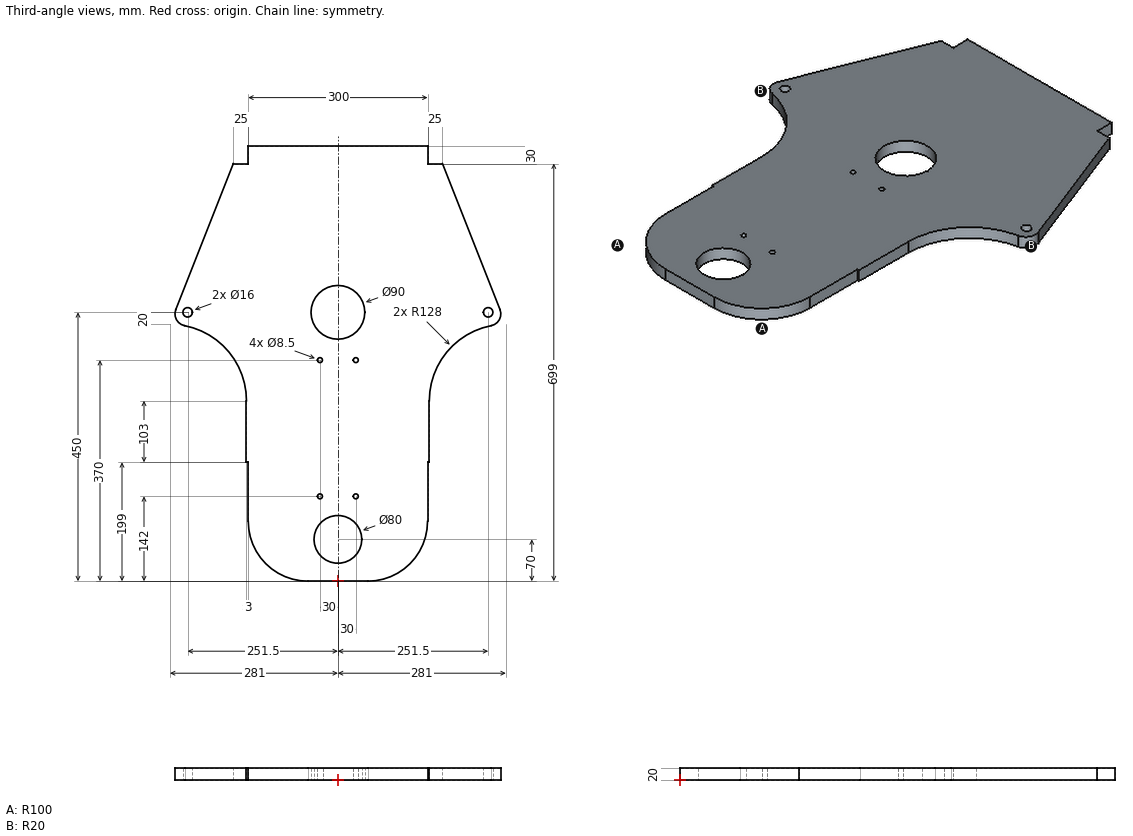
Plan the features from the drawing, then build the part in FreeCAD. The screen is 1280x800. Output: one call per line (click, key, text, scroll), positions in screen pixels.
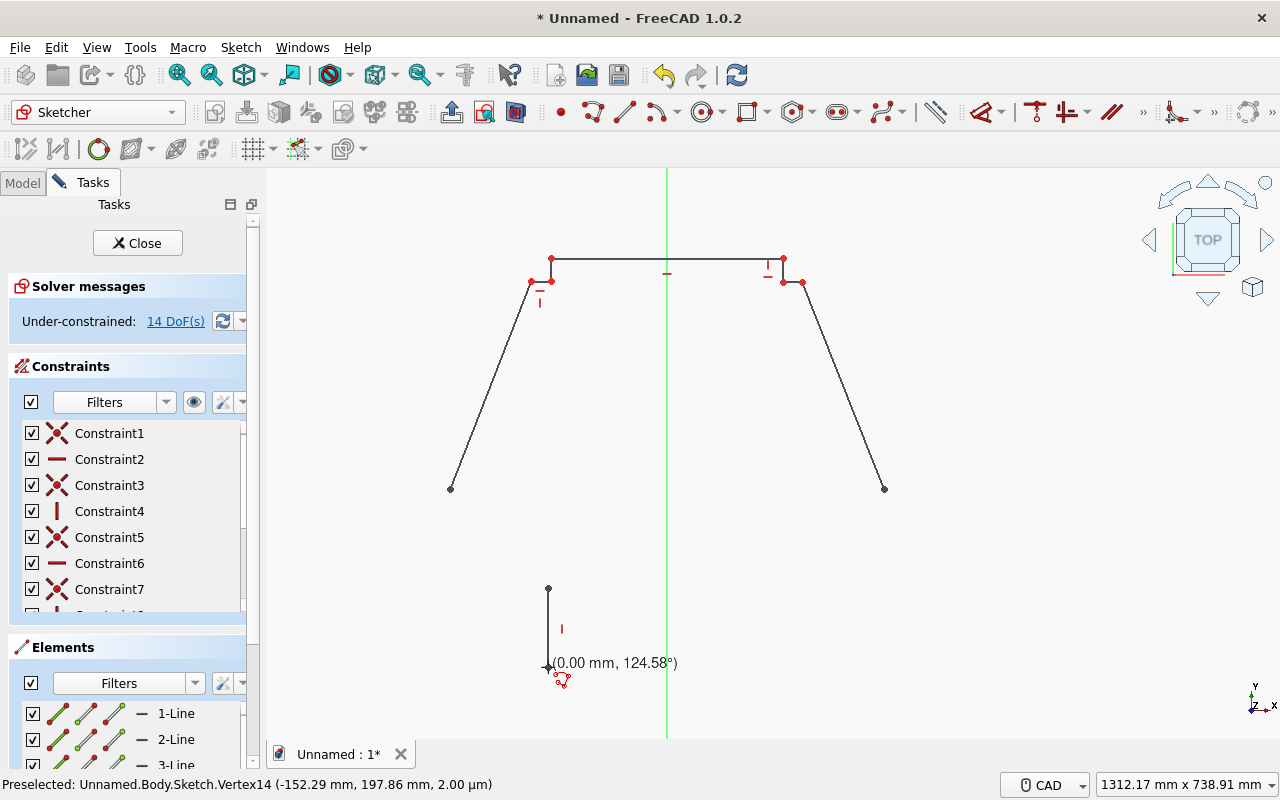
scroll(551, 667, up, 10)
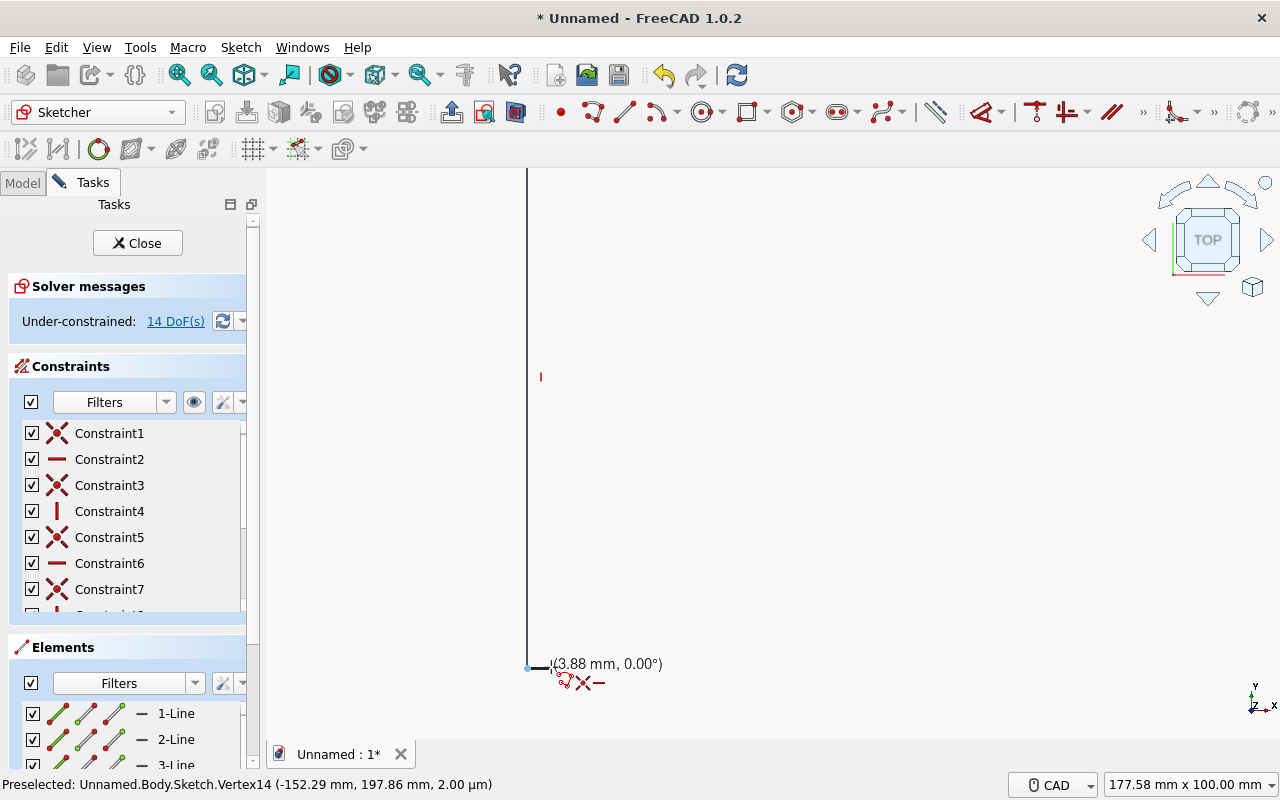
click(547, 661)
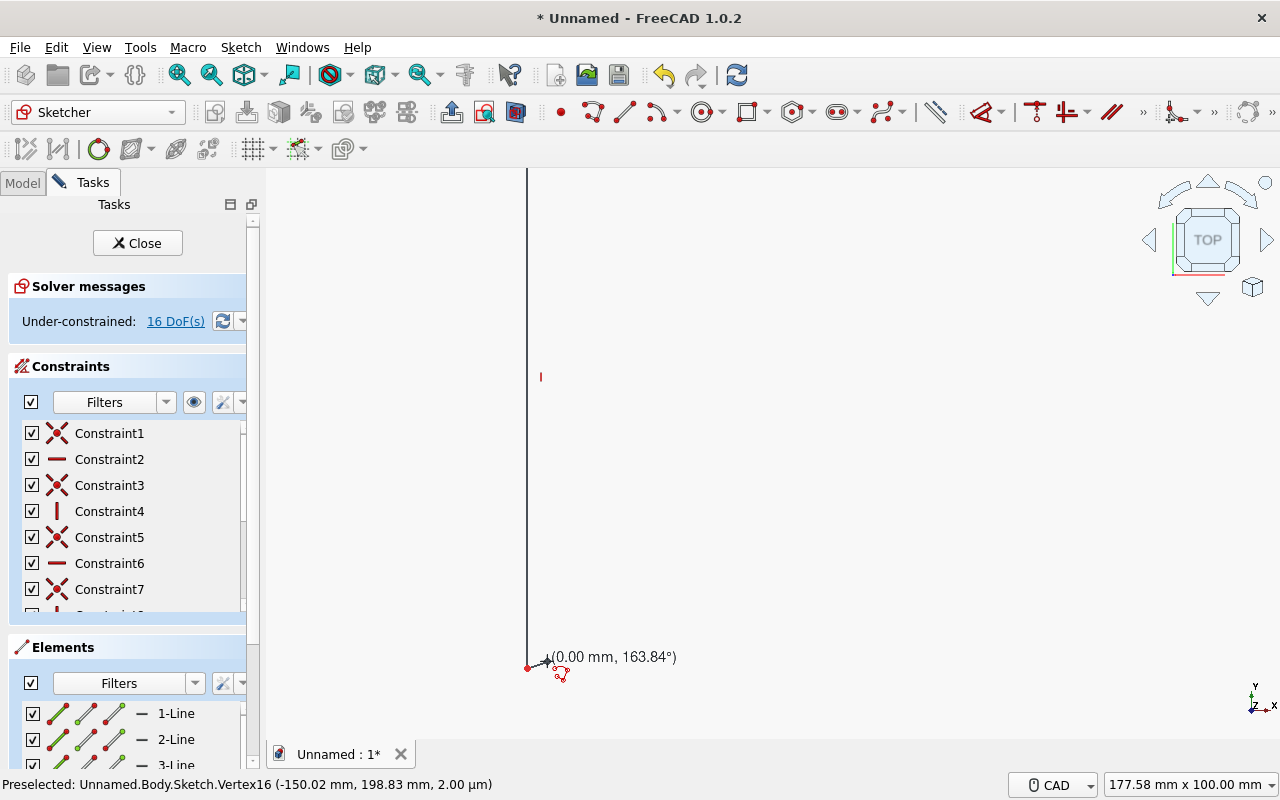
scroll(635, 527, down, 12)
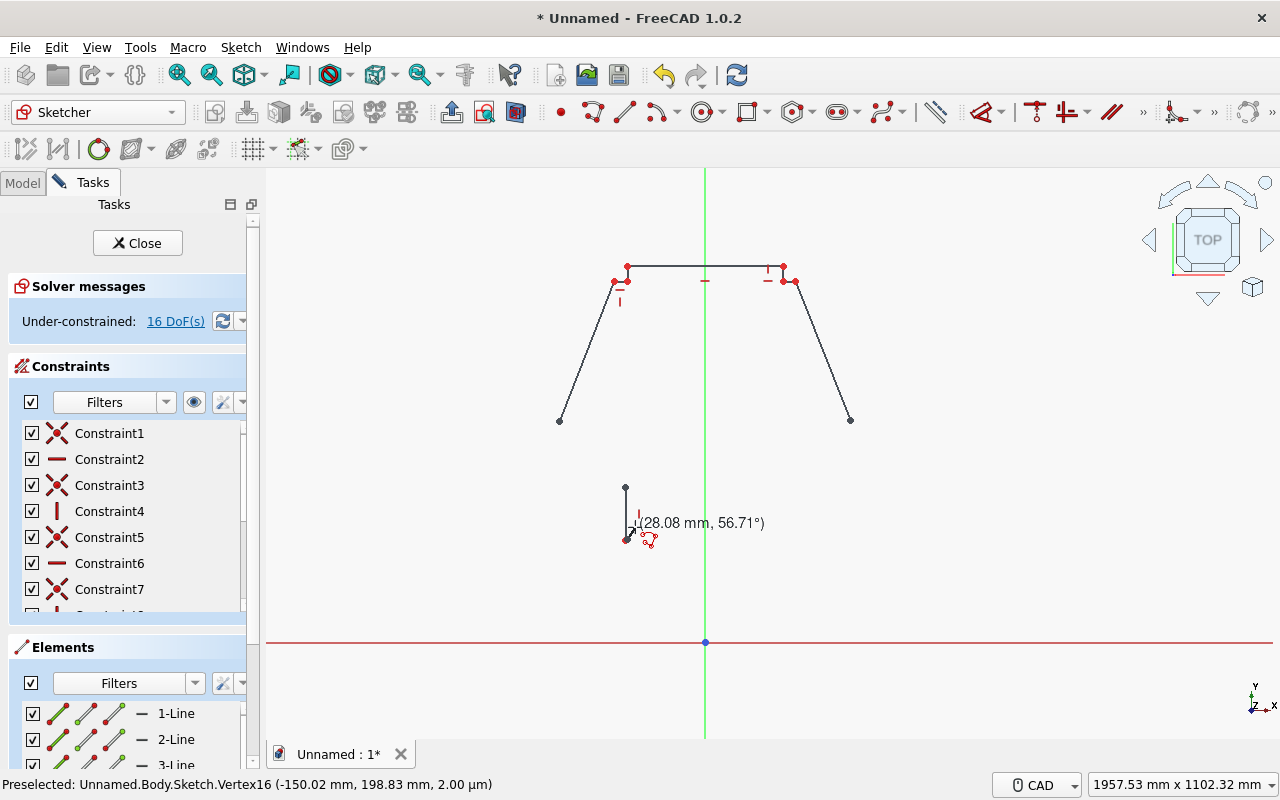
click(627, 643)
click(783, 634)
click(783, 540)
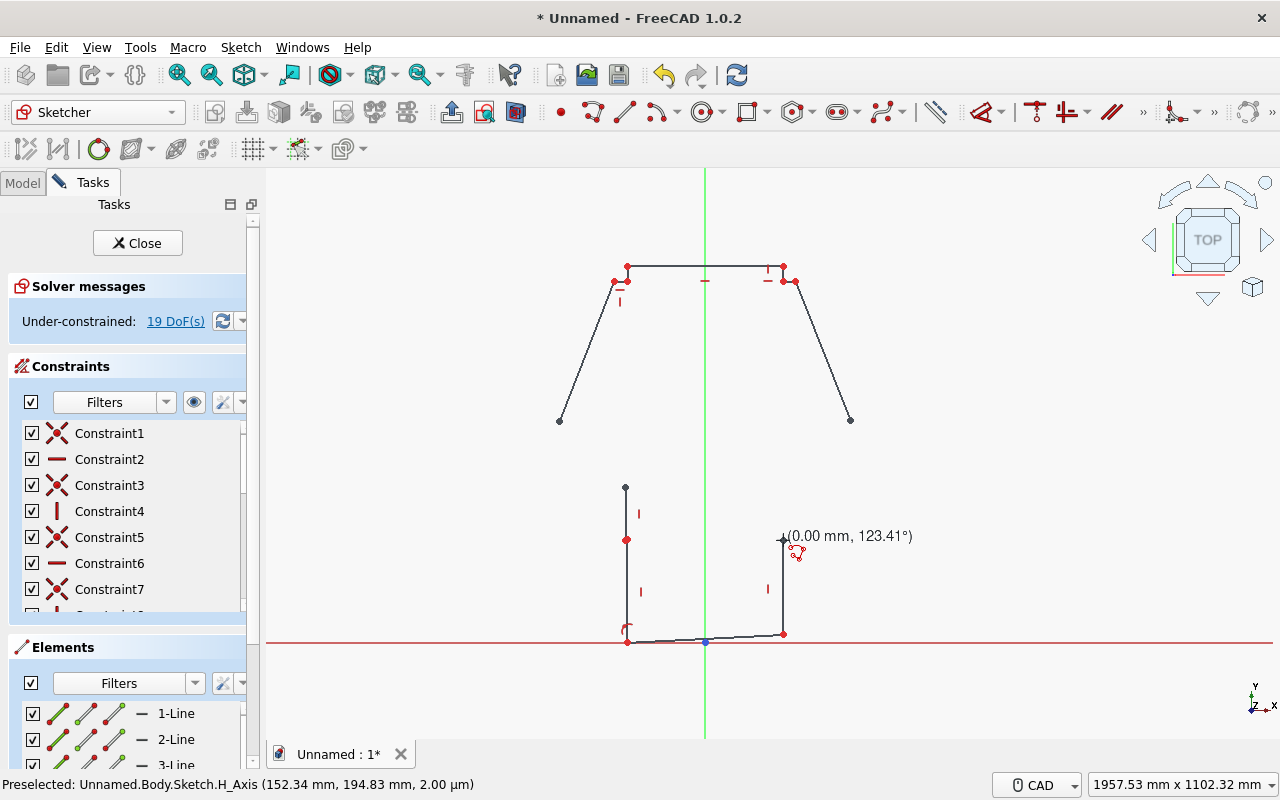
scroll(784, 540, up, 12)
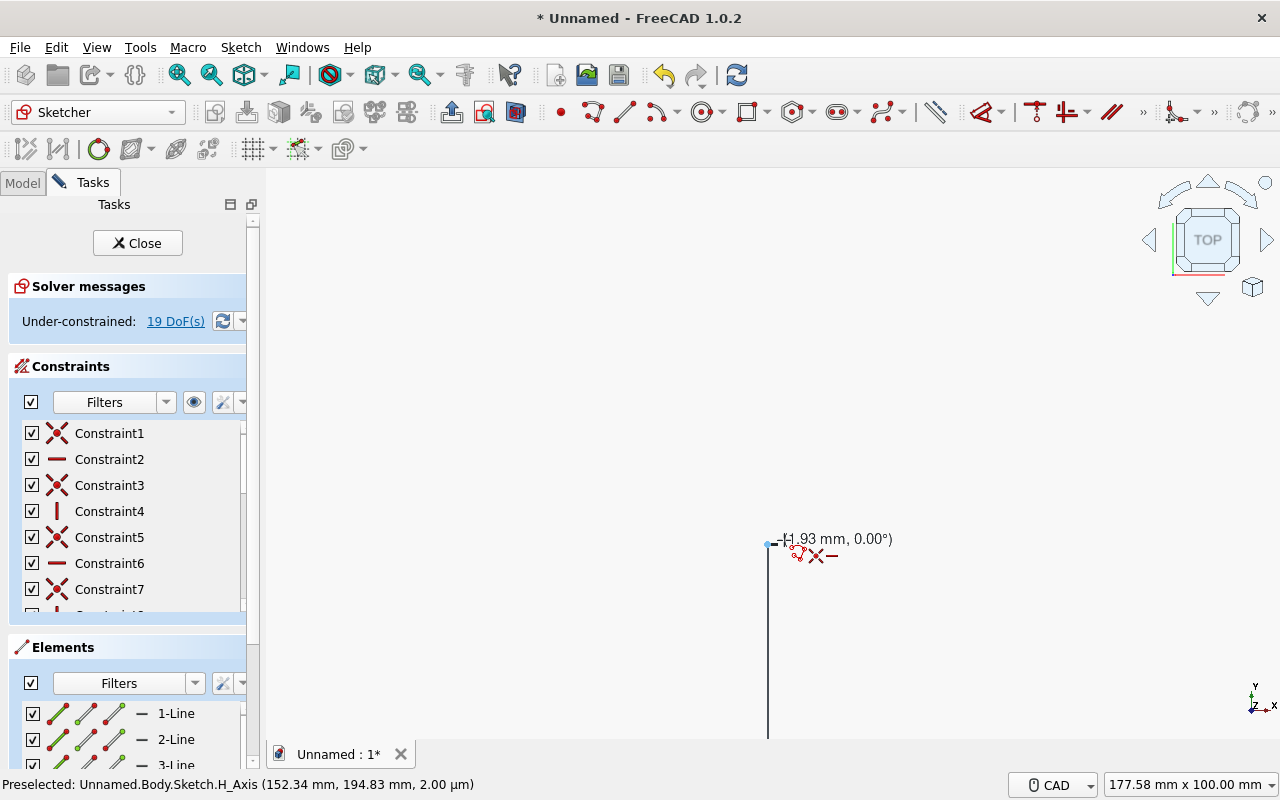
click(783, 533)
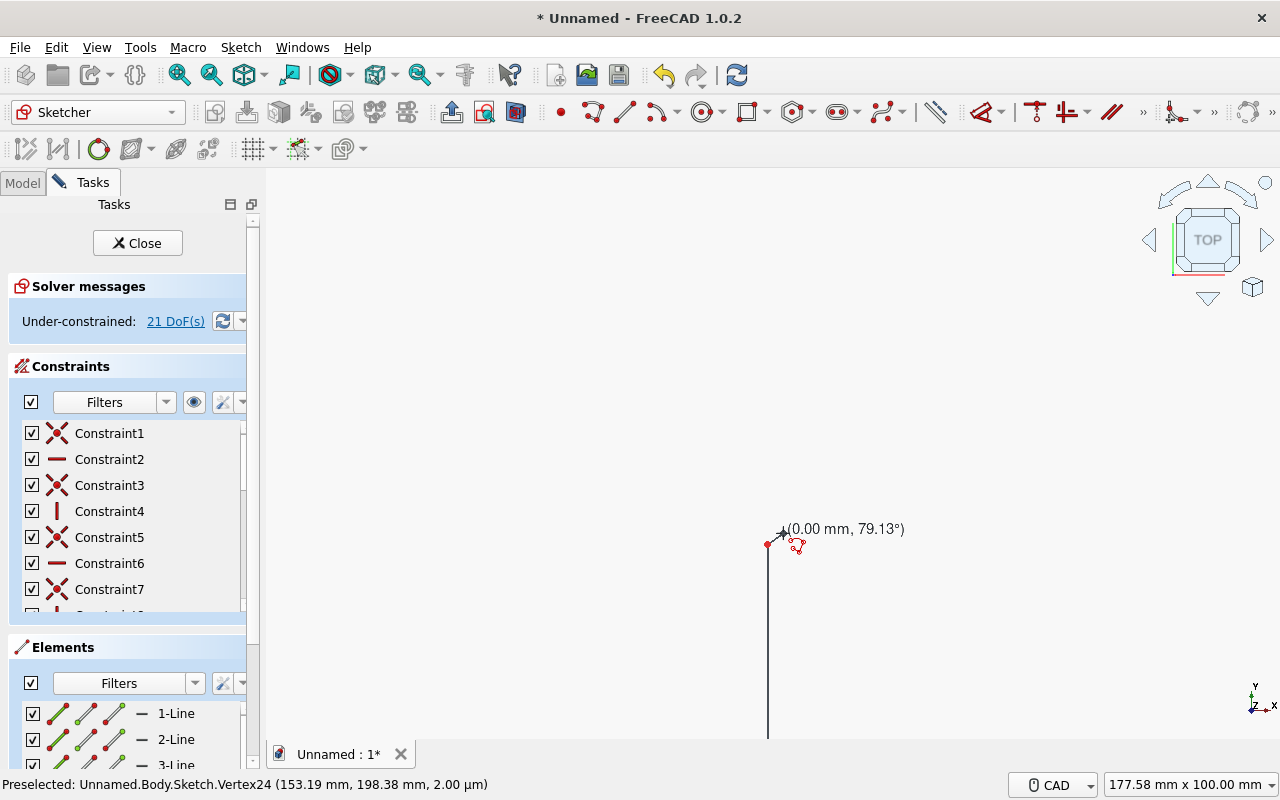
scroll(784, 540, down, 12)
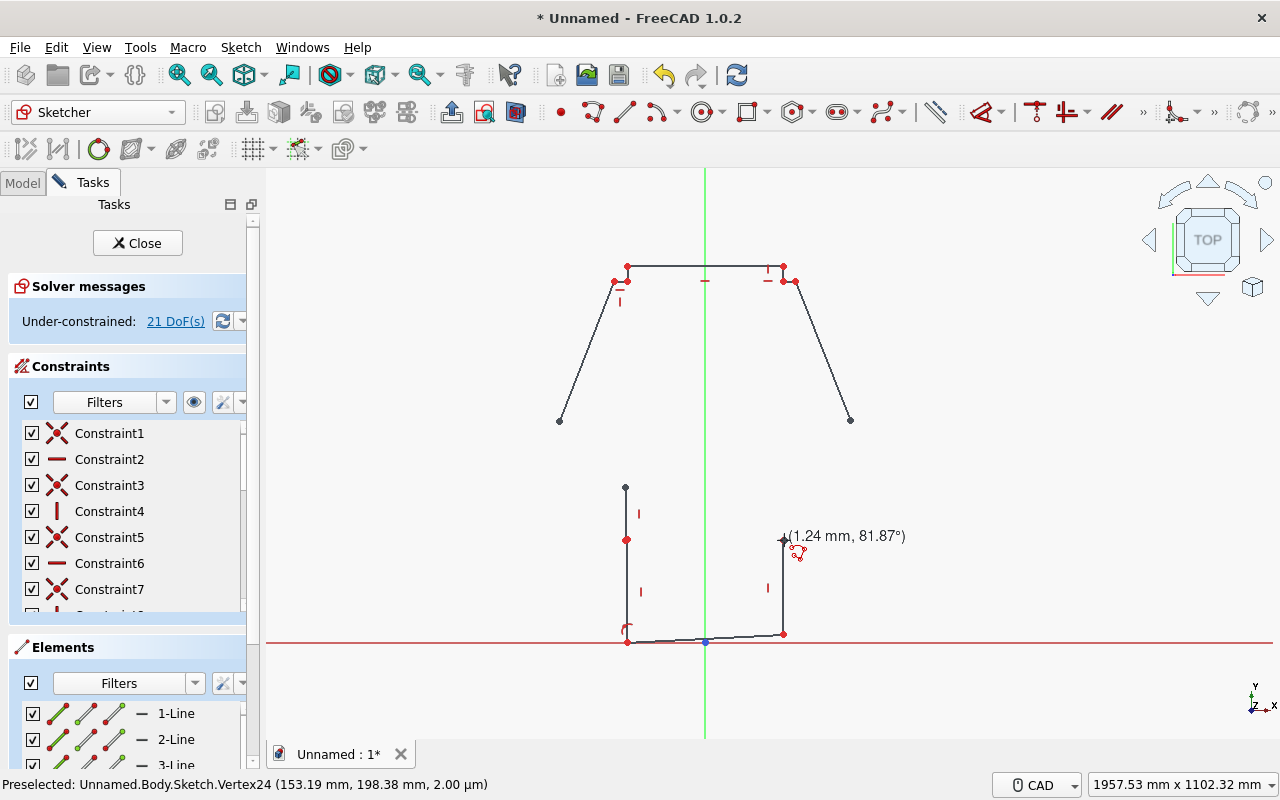
click(784, 486)
right_click(784, 486)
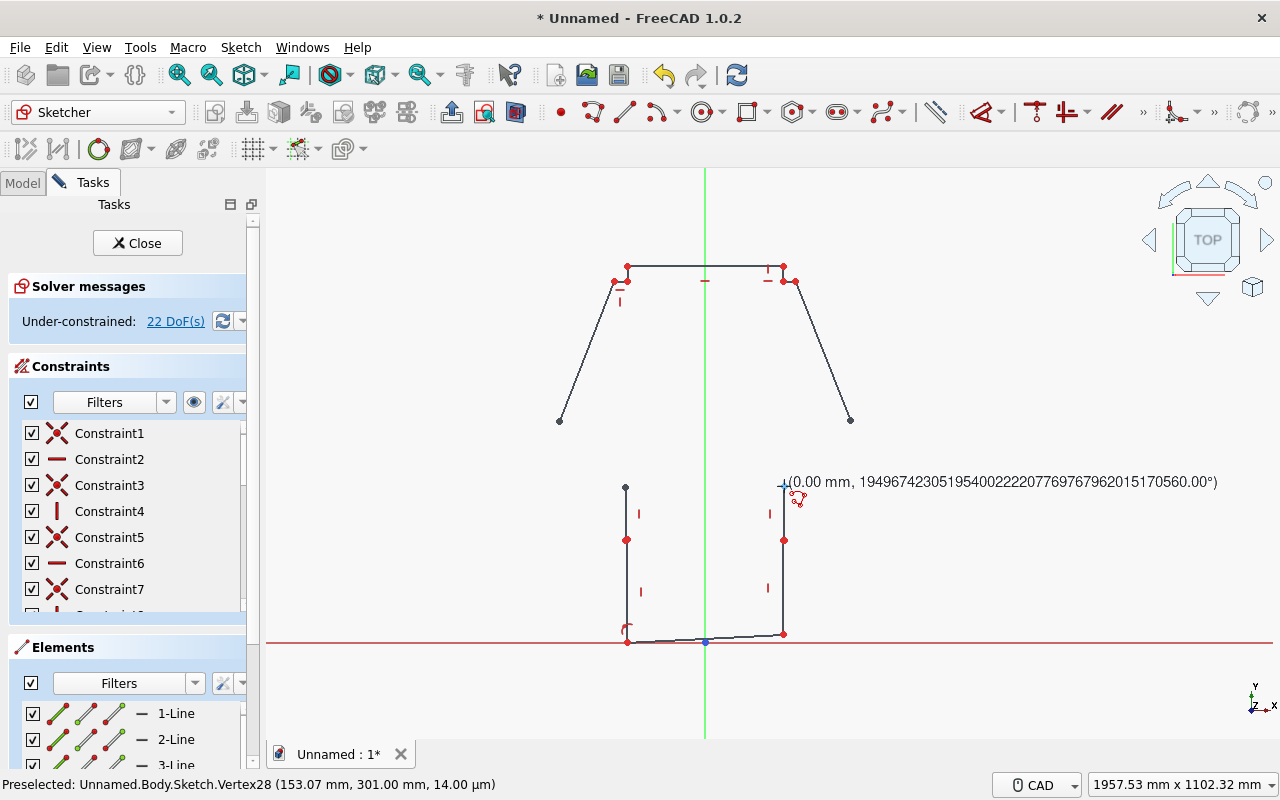
key(g)
key(3)
key(a)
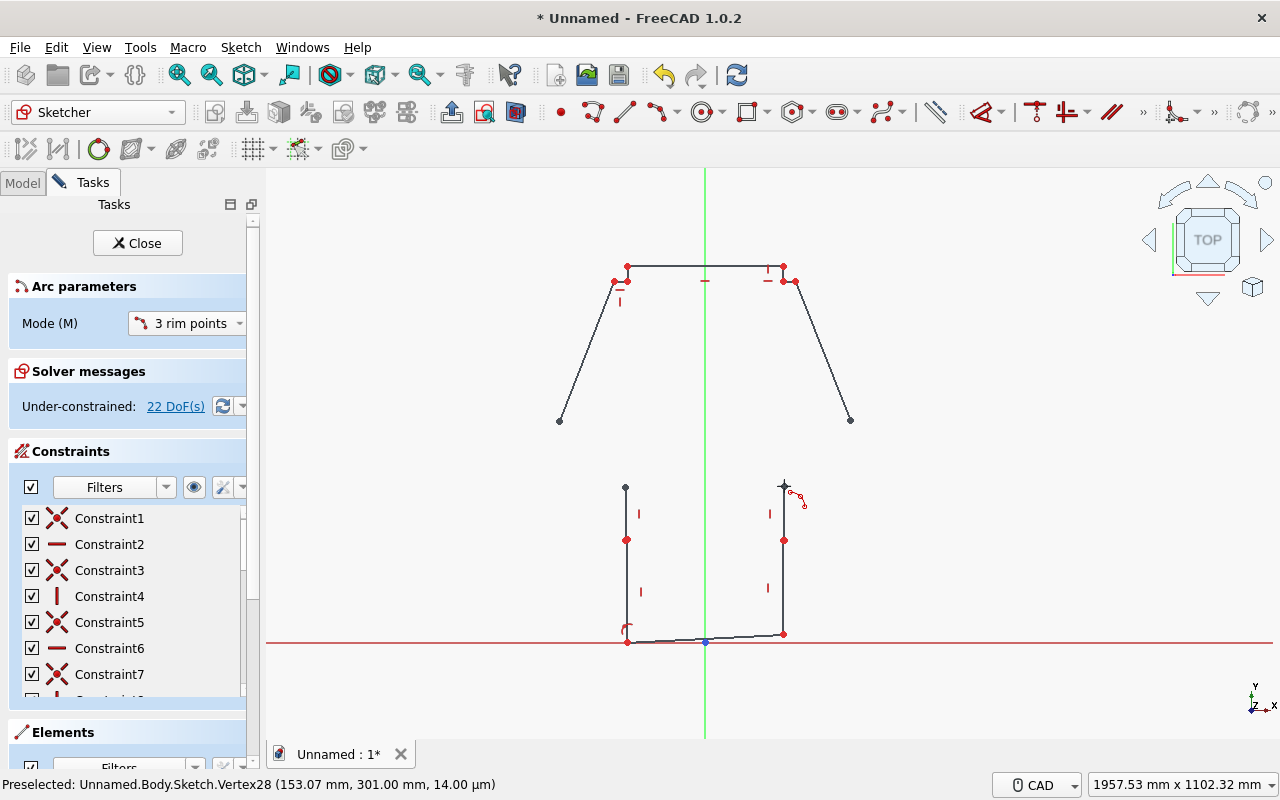
click(560, 421)
click(626, 487)
click(606, 440)